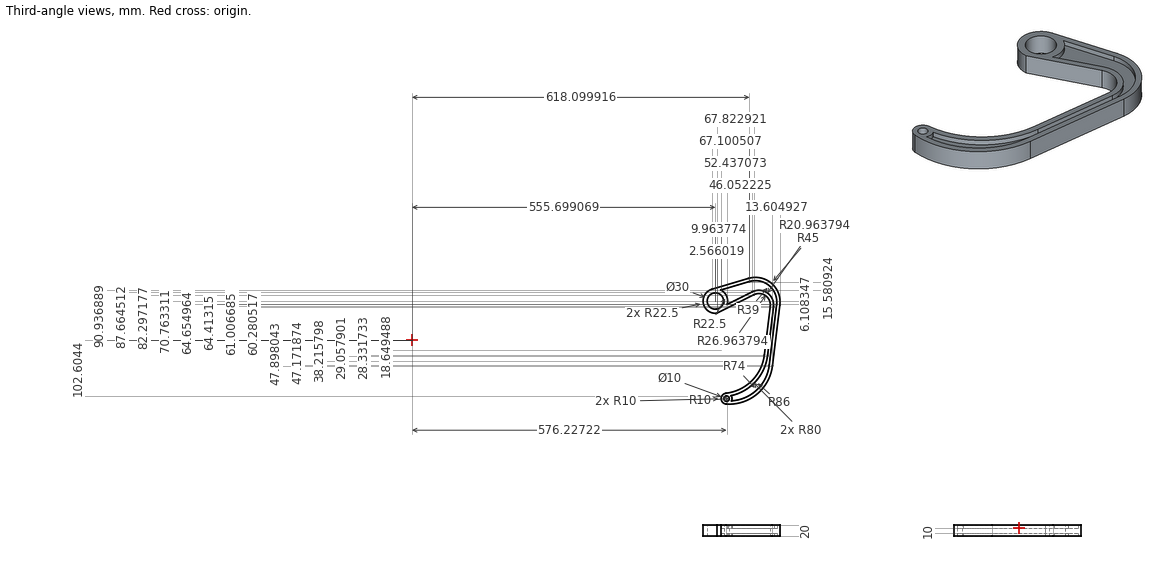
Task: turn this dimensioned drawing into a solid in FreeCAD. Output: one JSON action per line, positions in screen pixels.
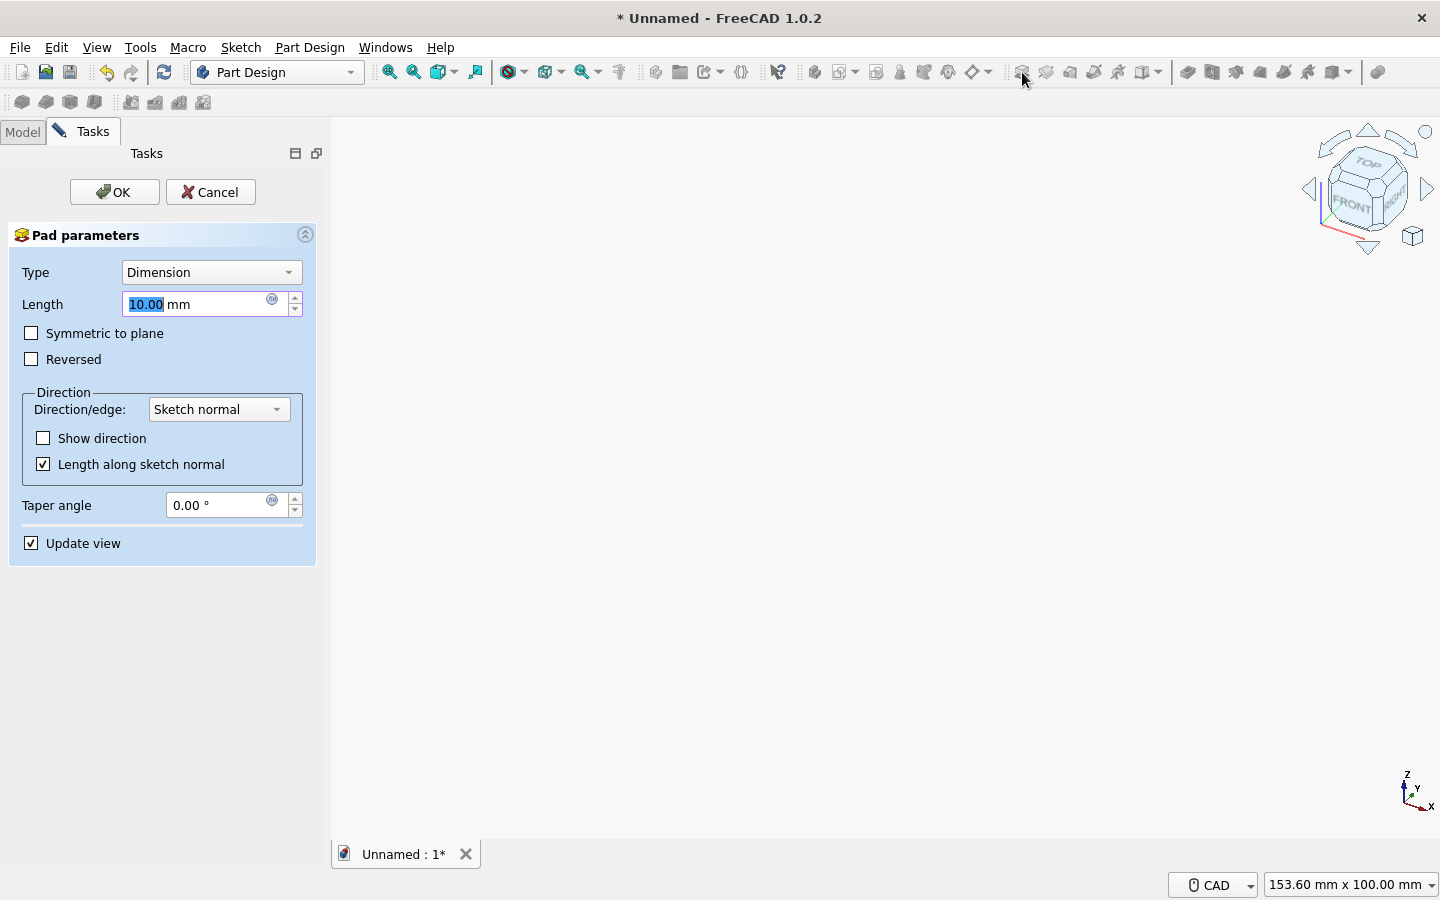
{"action": "type", "text": "10"}
{"action": "key", "text": "Tab"}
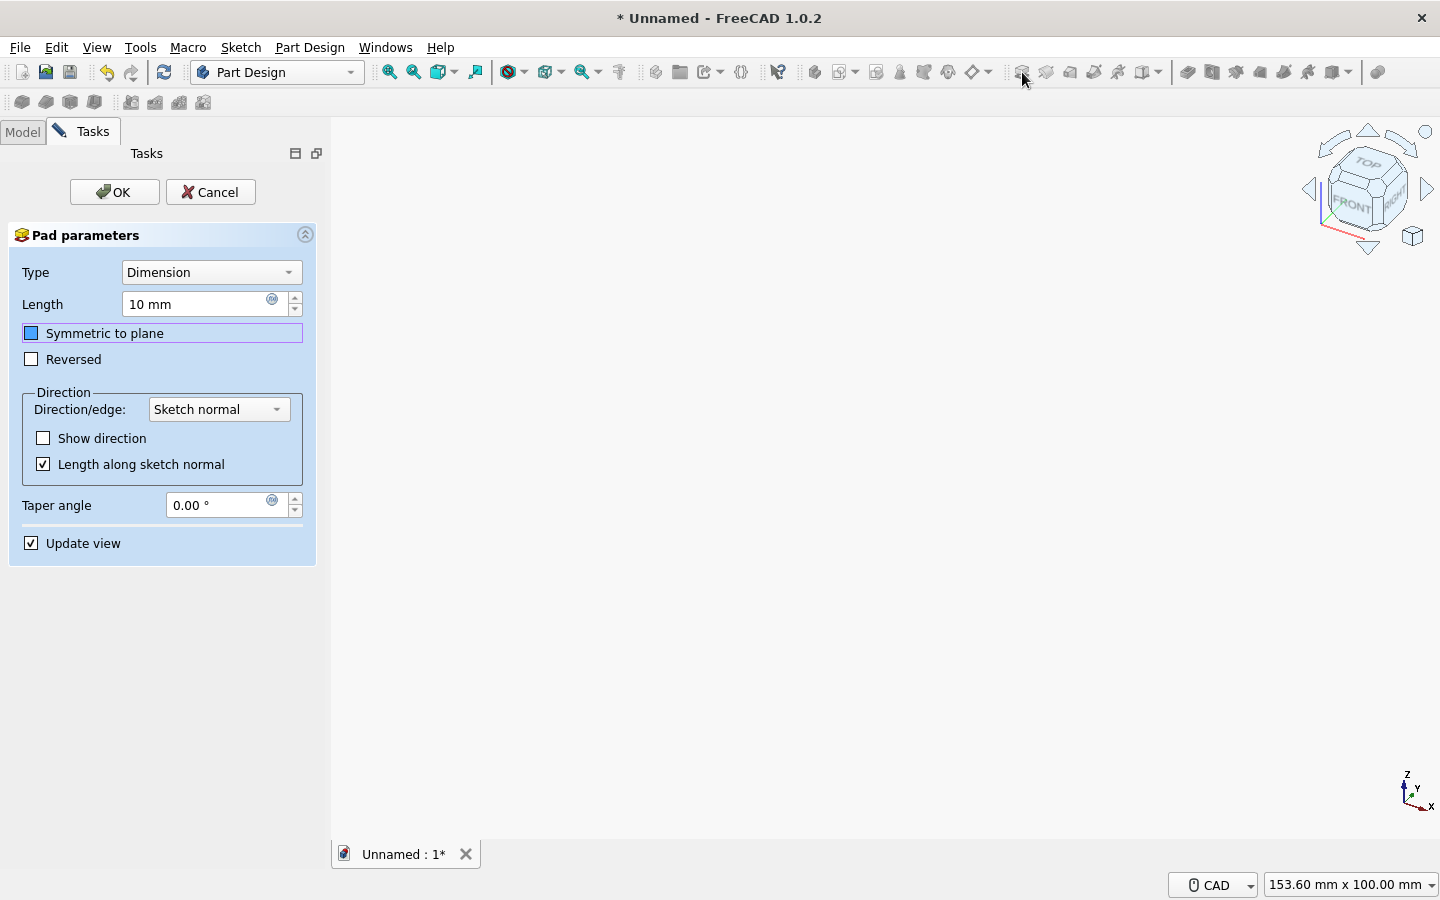
{"action": "left_click", "coordinate": [30, 359]}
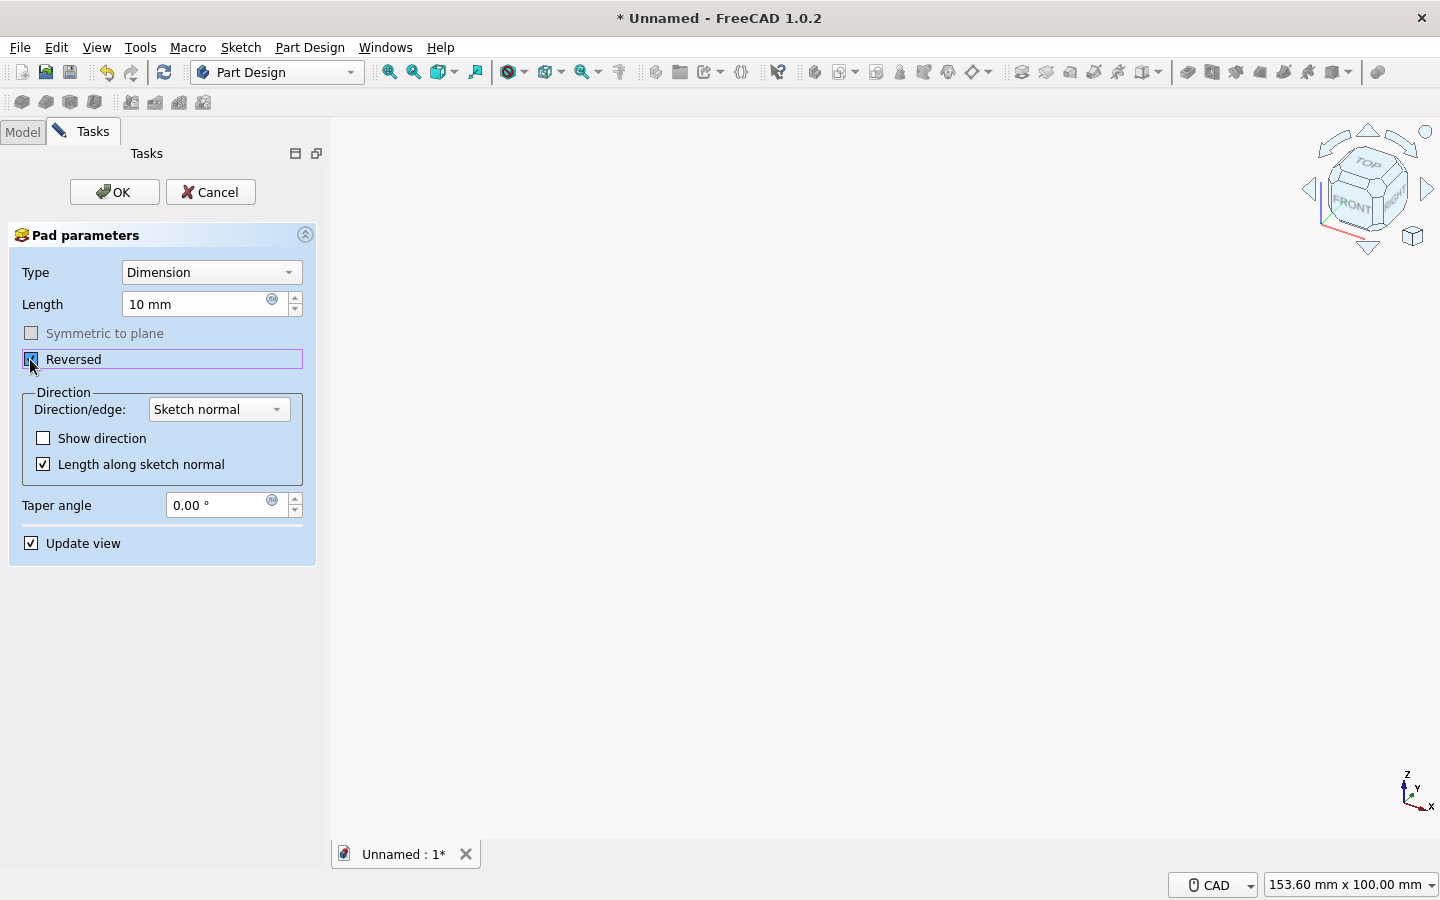
{"action": "left_click", "coordinate": [115, 192]}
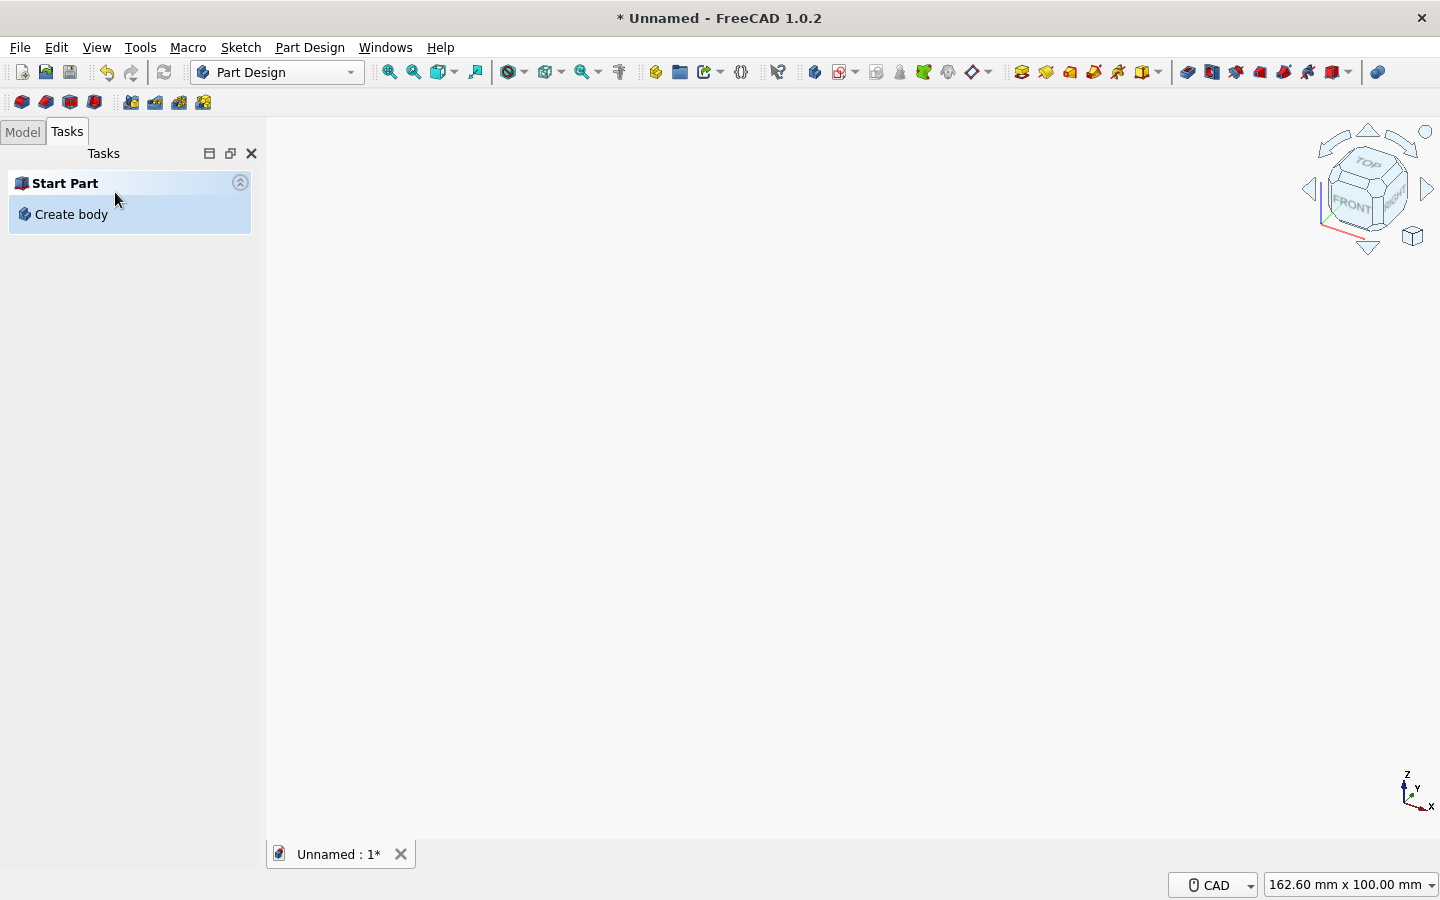
{"action": "left_click", "coordinate": [390, 72]}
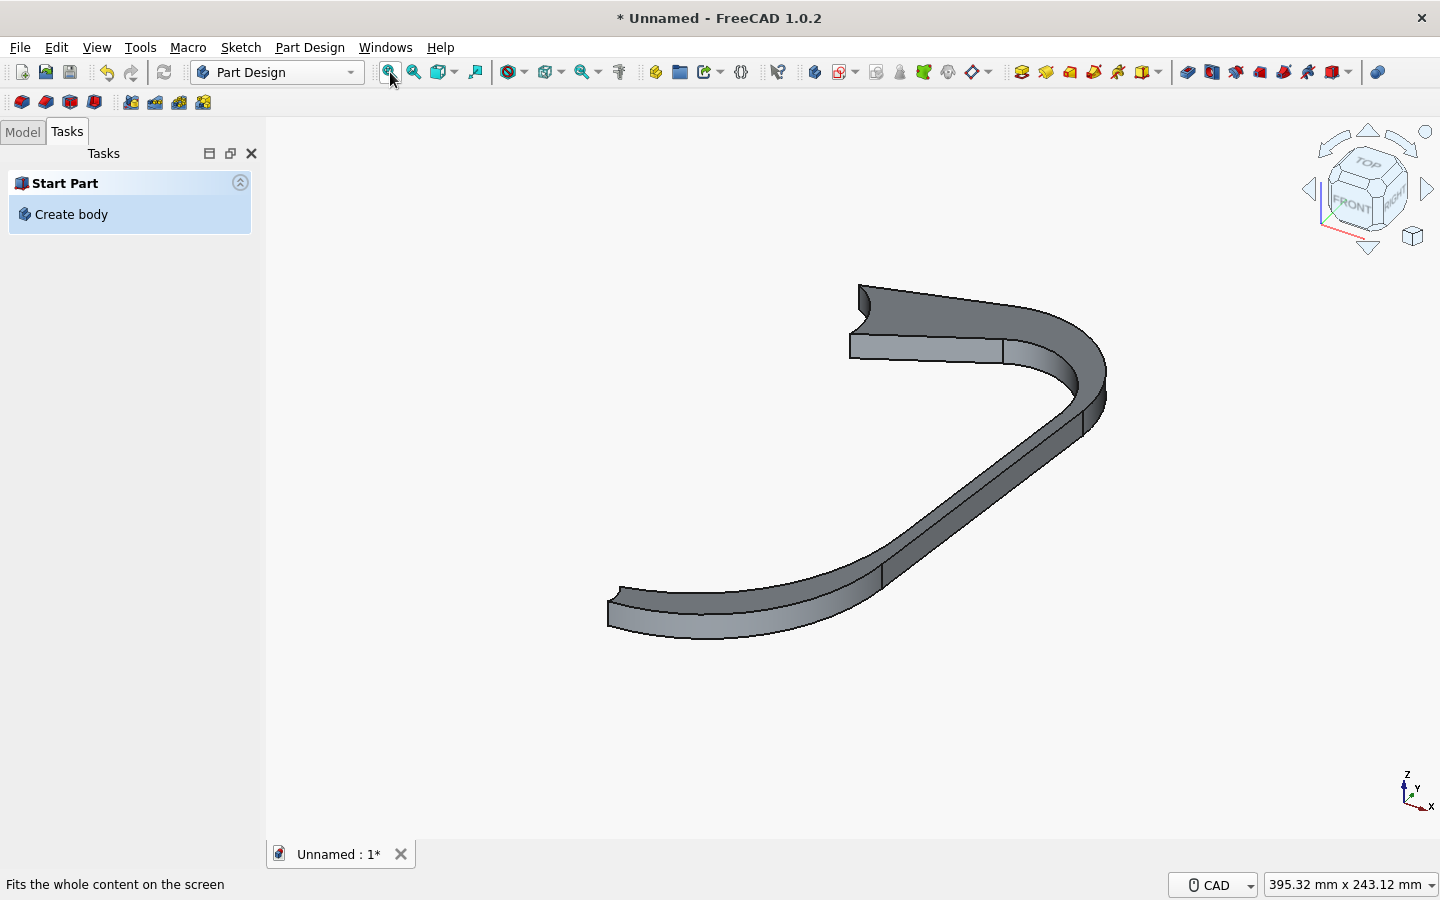
{"action": "left_click", "coordinate": [23, 131]}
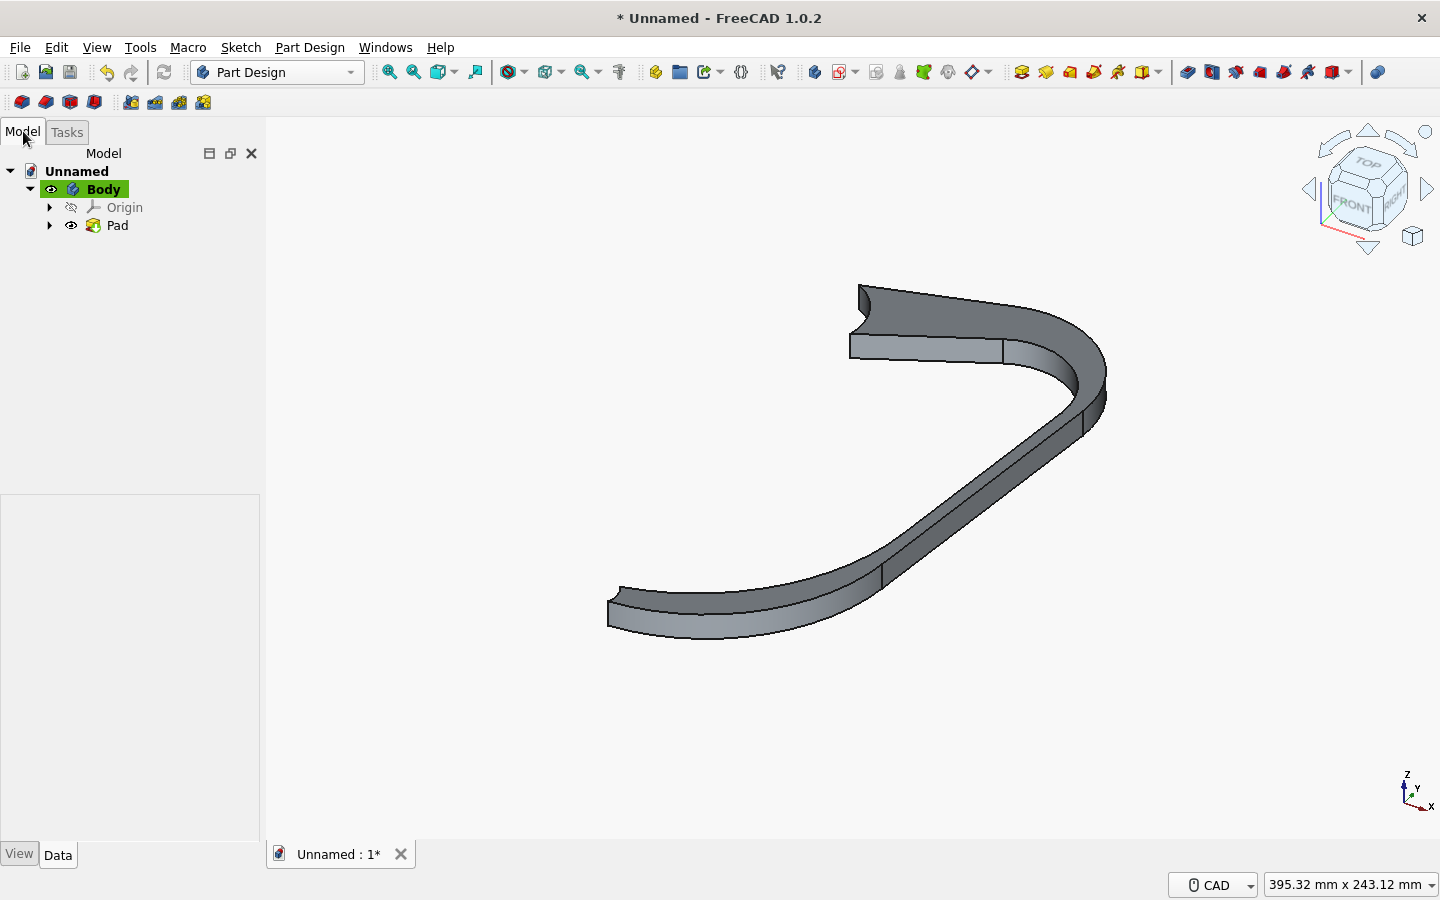
{"action": "left_click", "coordinate": [50, 207]}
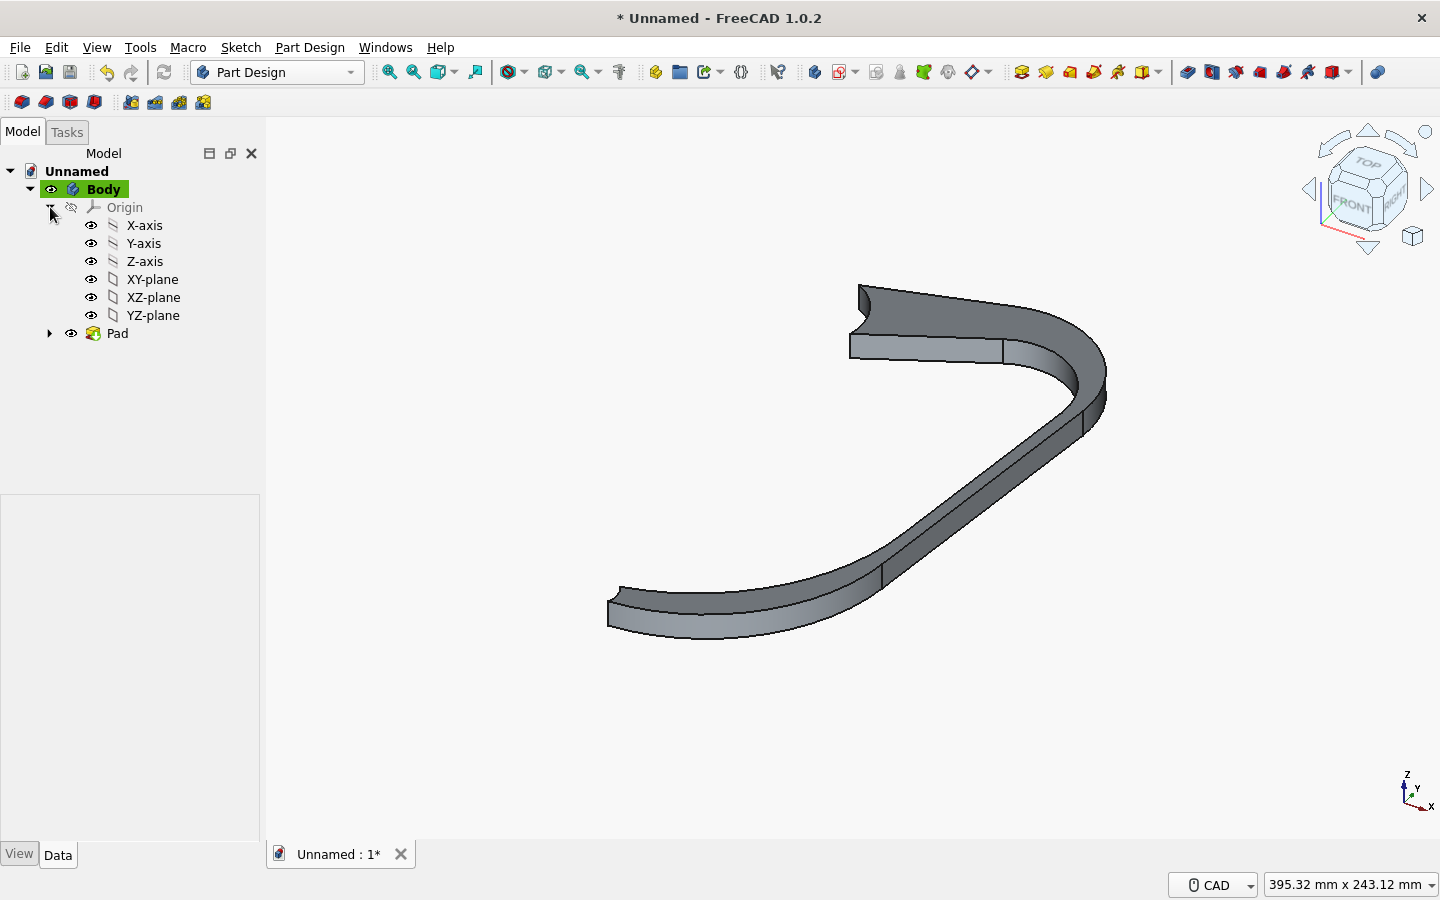
{"action": "left_click", "coordinate": [136, 279]}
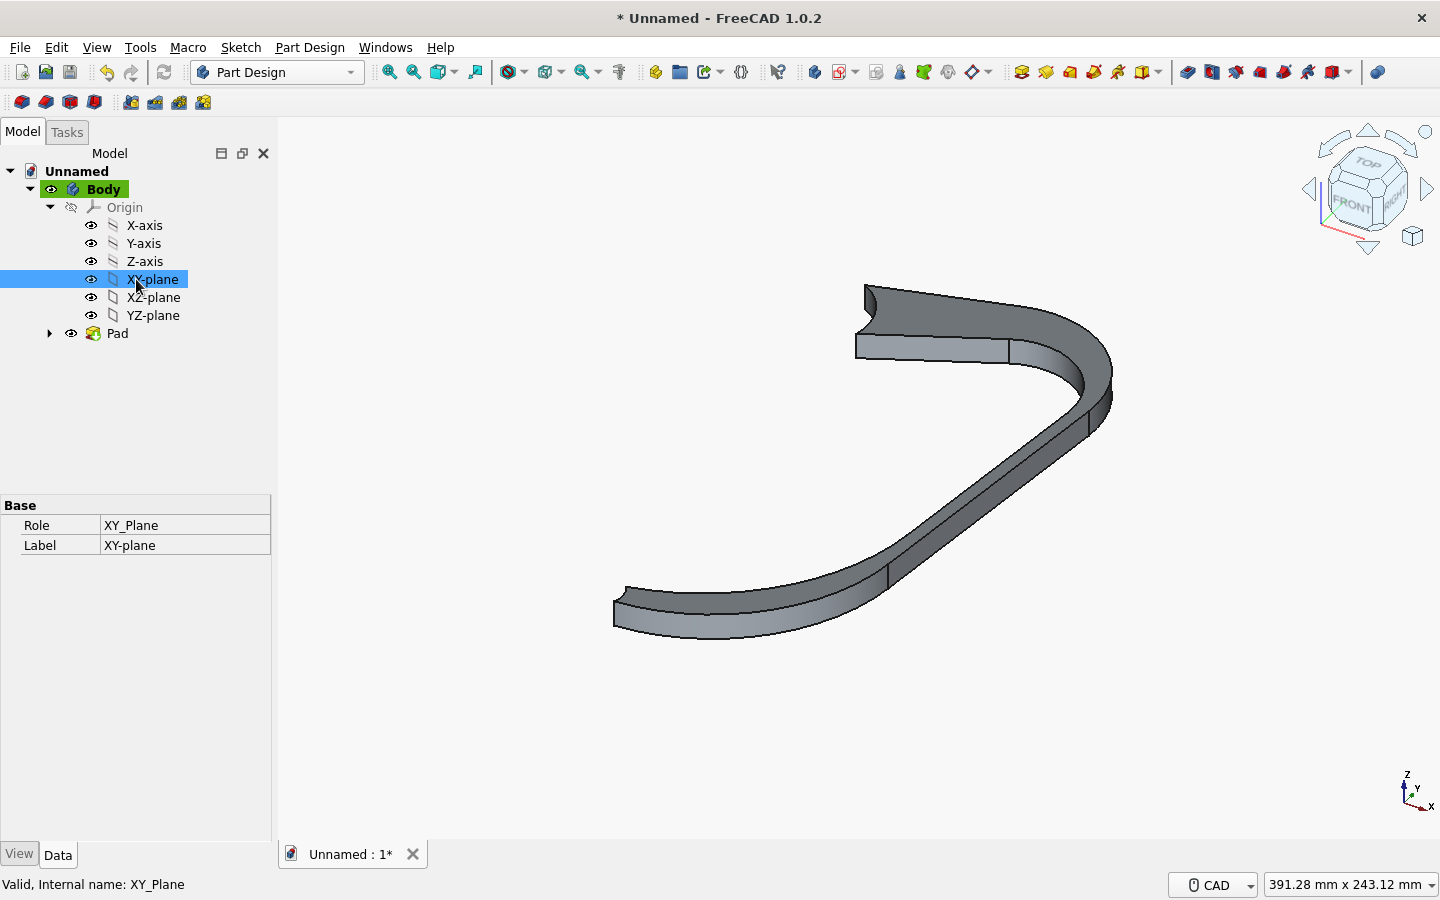
{"action": "left_click", "coordinate": [972, 72]}